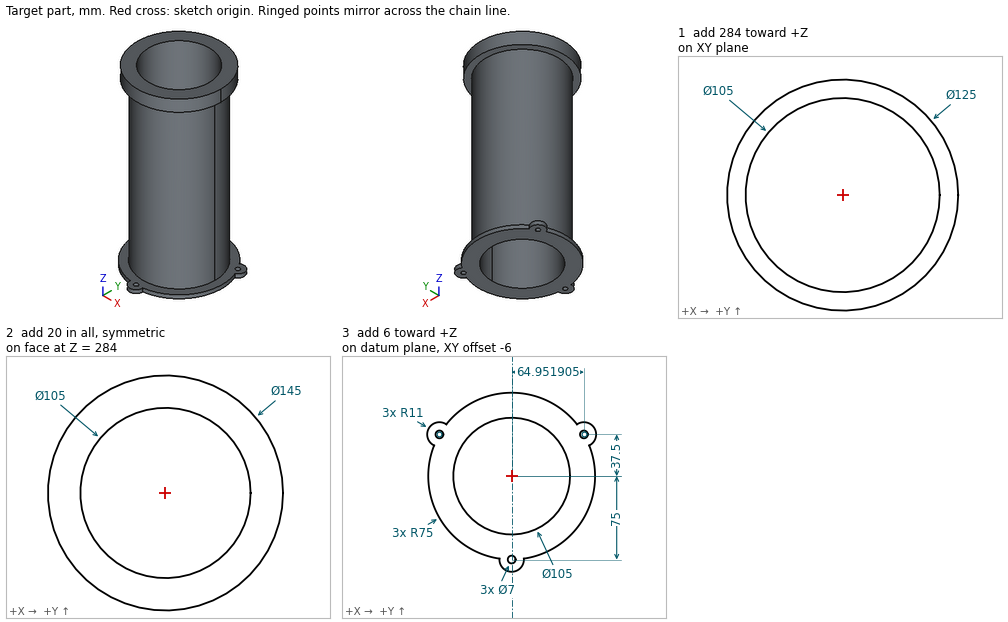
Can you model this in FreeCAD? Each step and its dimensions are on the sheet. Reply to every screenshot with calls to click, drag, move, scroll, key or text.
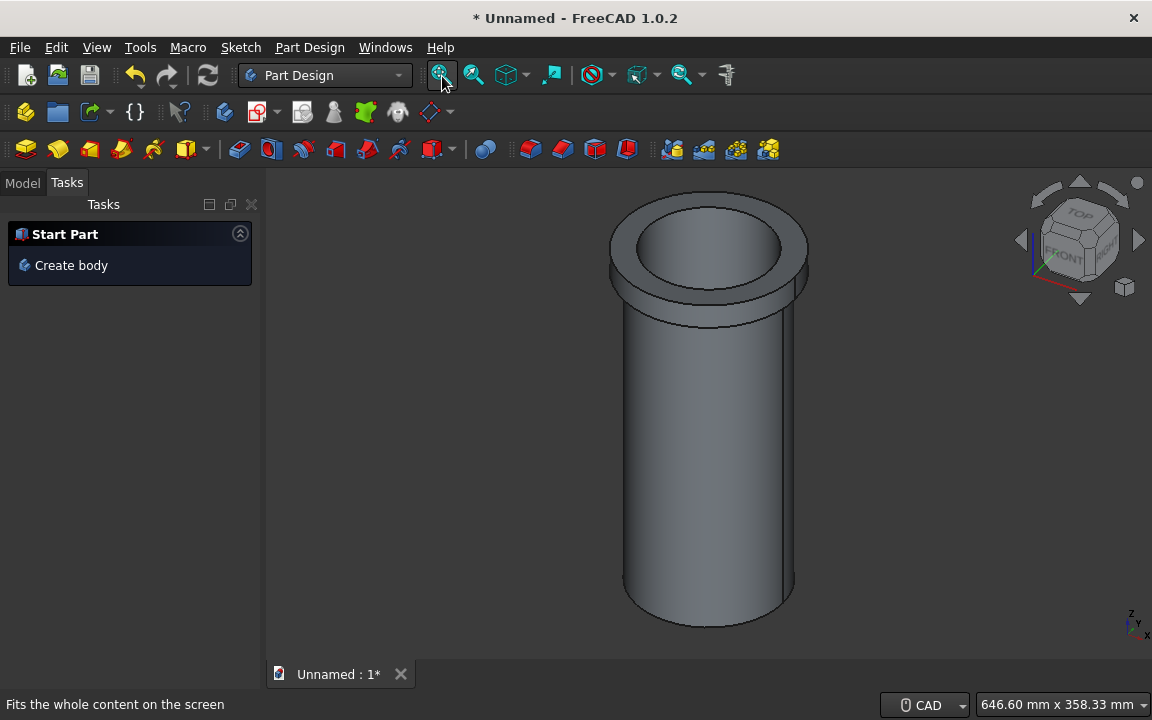
click(23, 182)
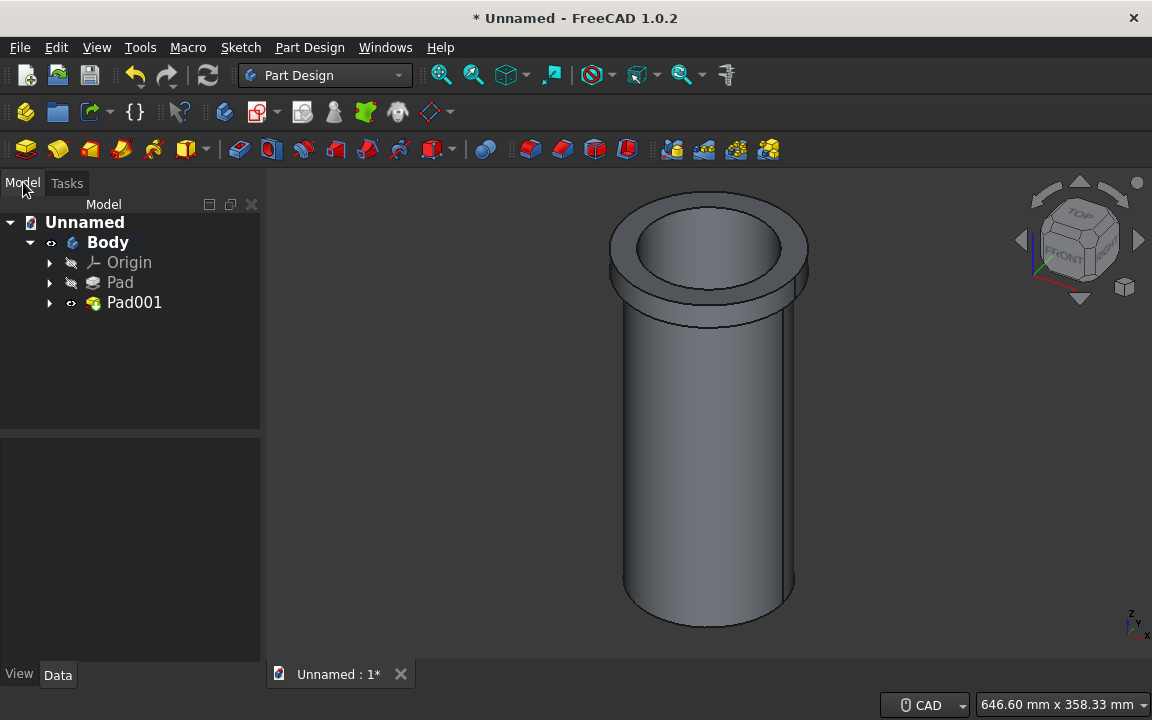
click(50, 263)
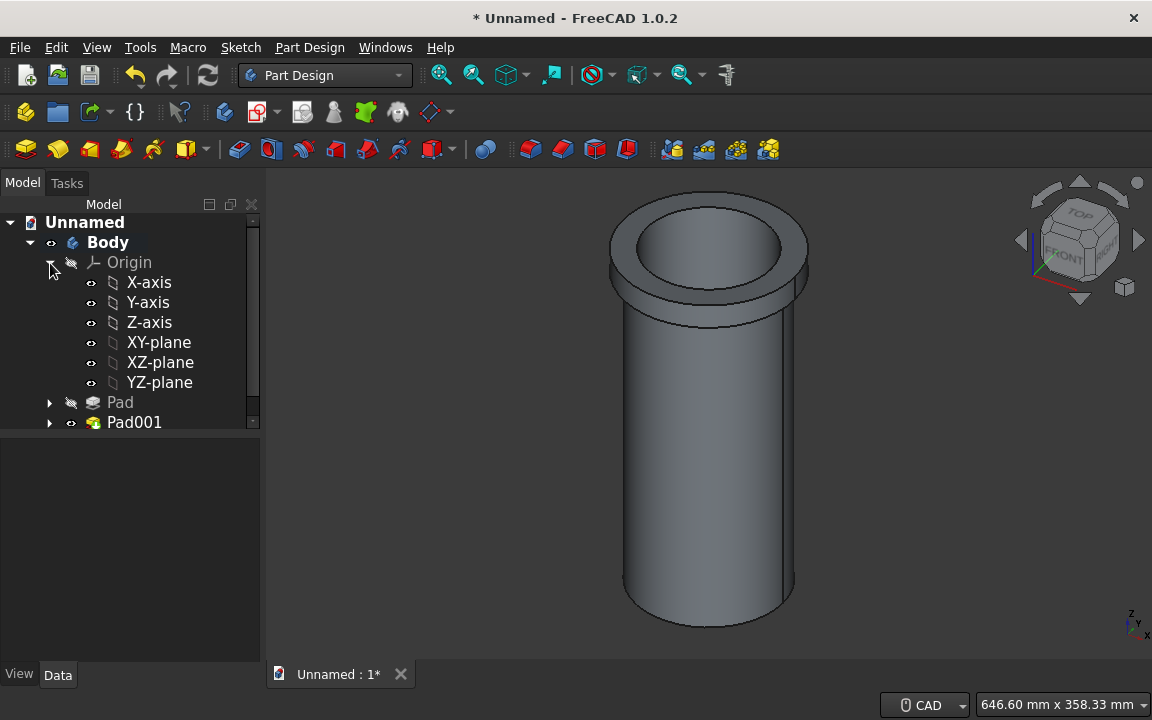
click(136, 343)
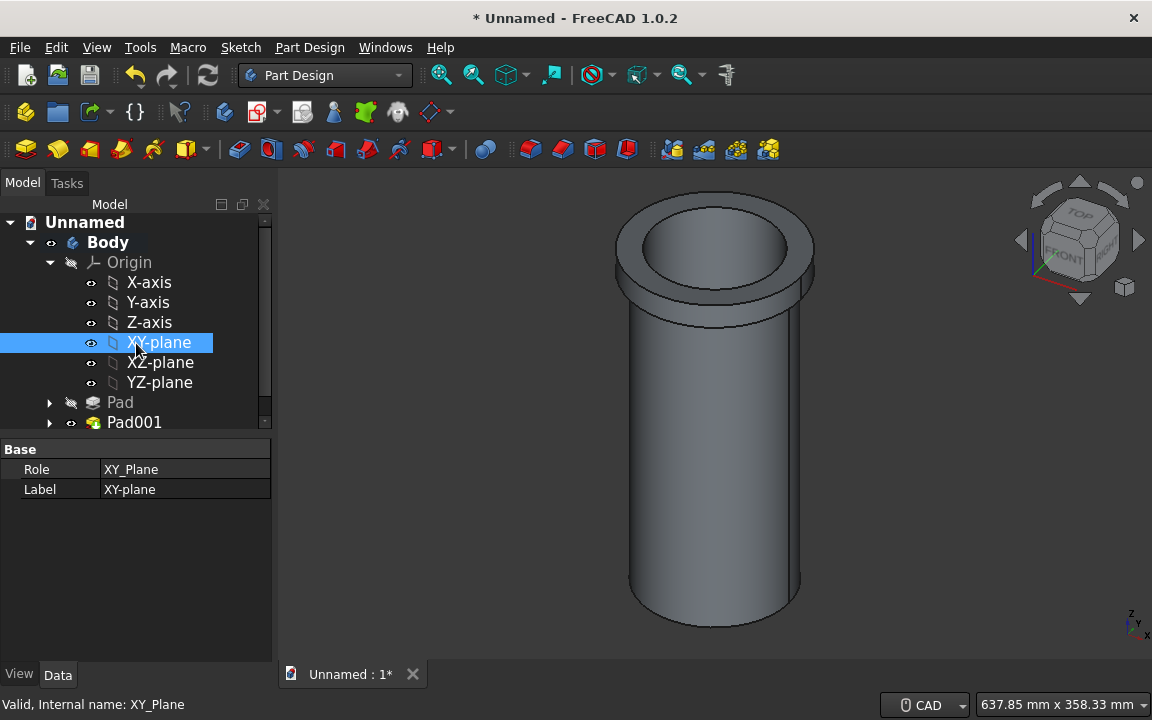
click(430, 112)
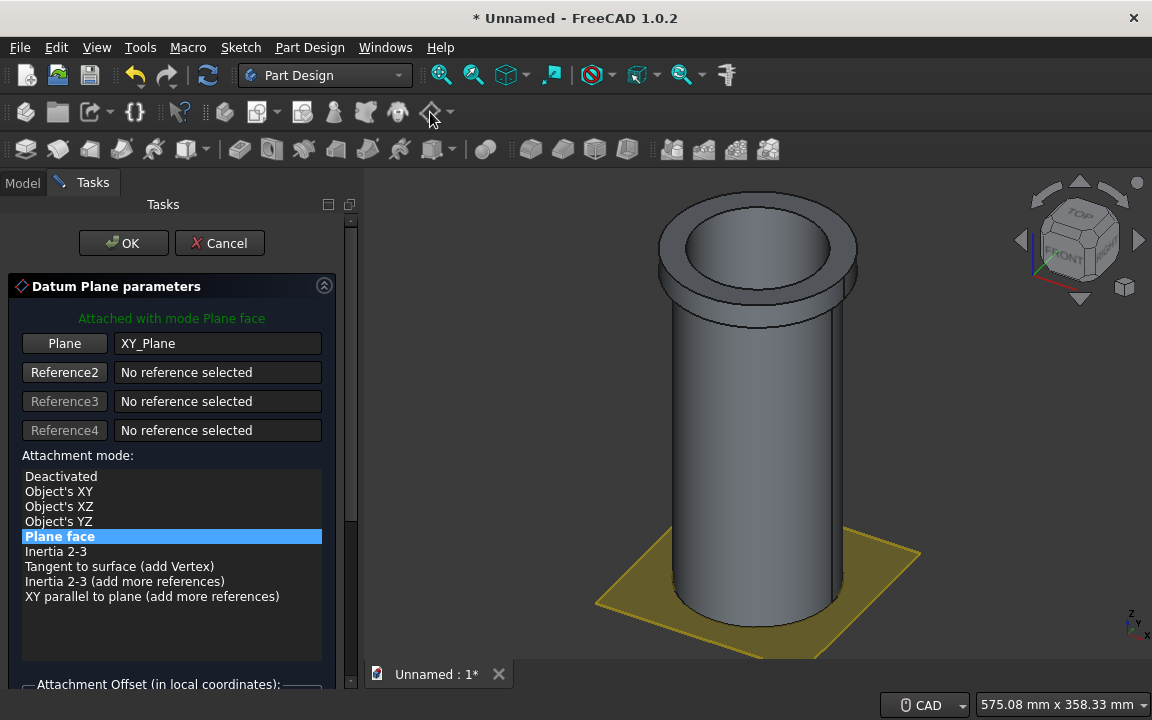
scroll(351, 451, down, 3)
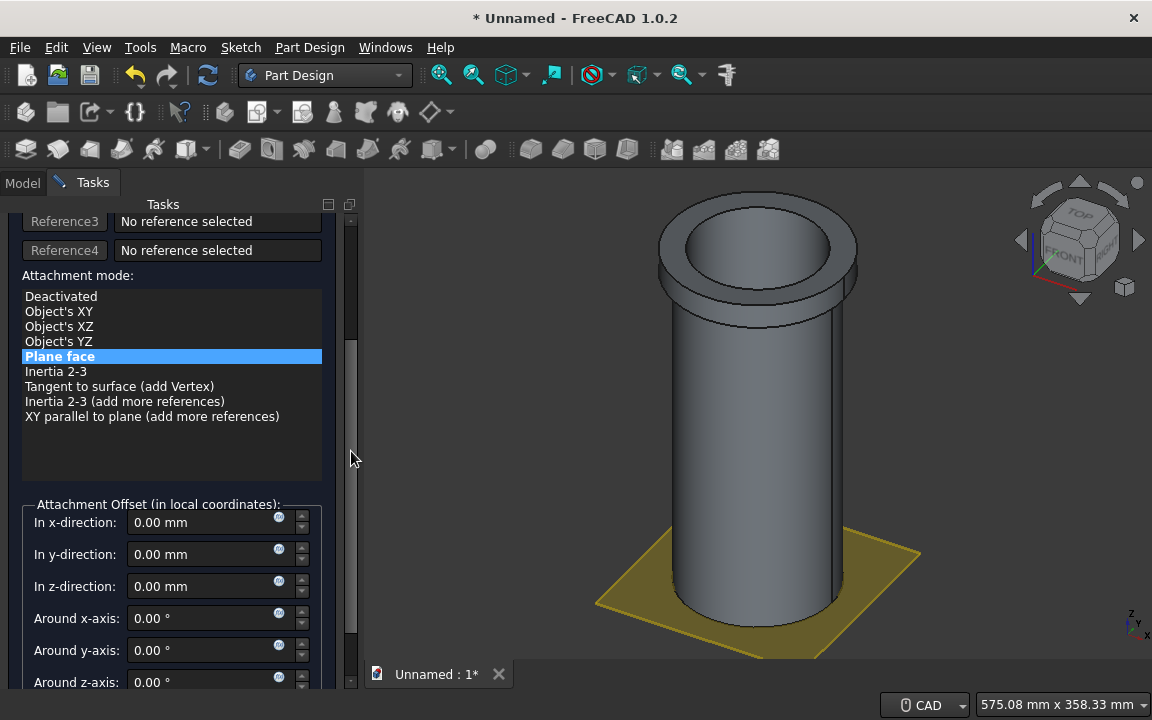
triple_click(210, 586)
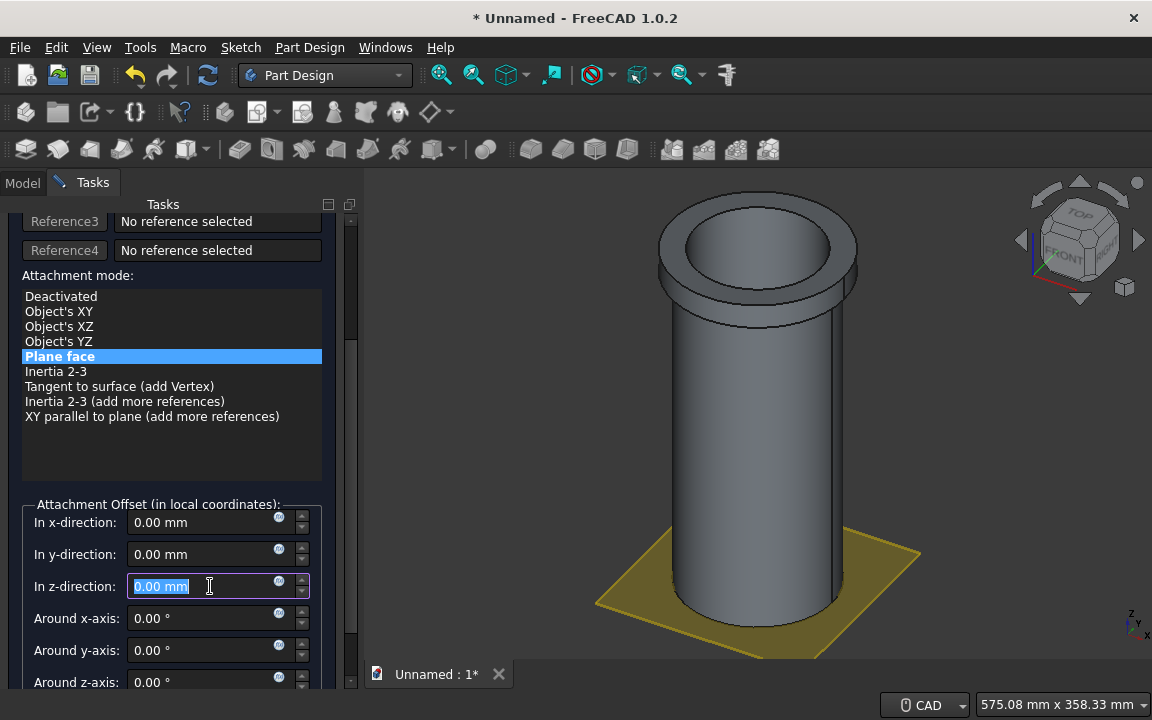
text(-6)
key(Tab)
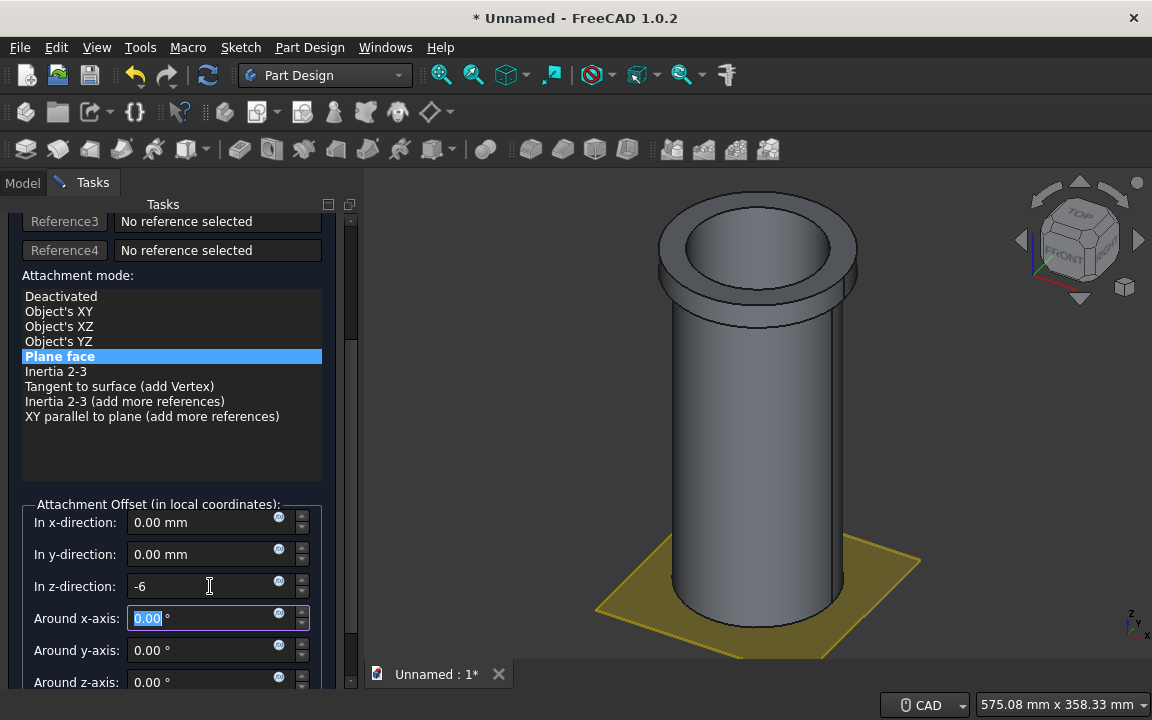
scroll(351, 451, up, 4)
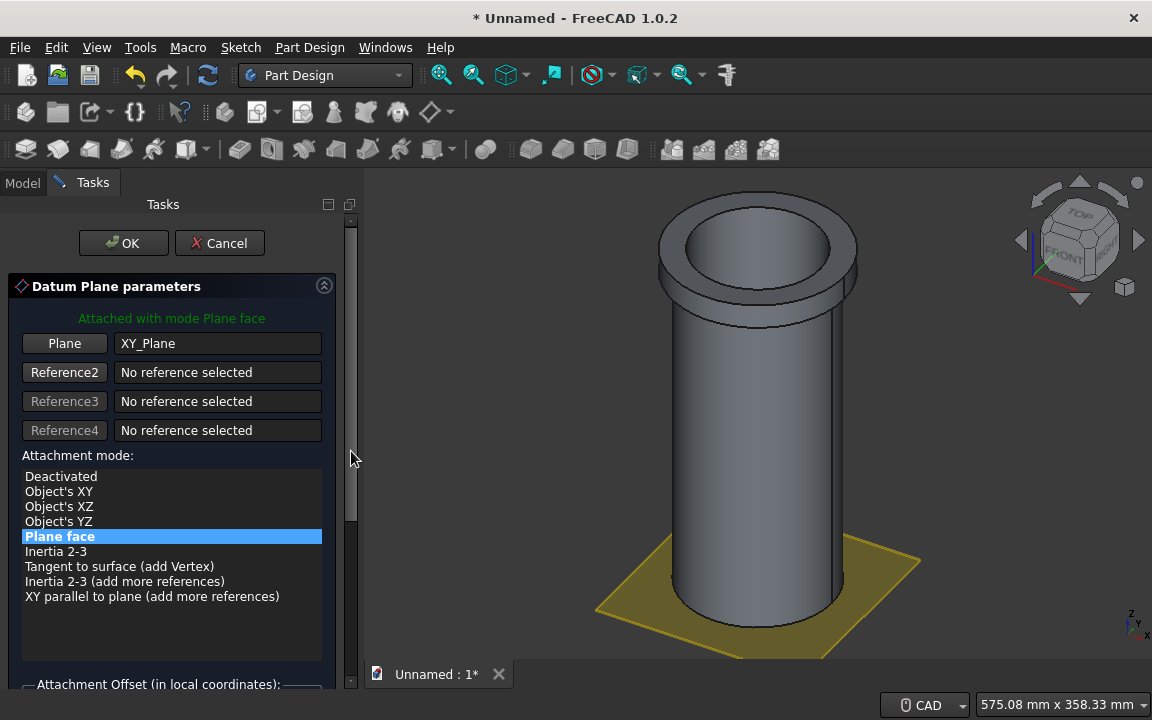
click(124, 243)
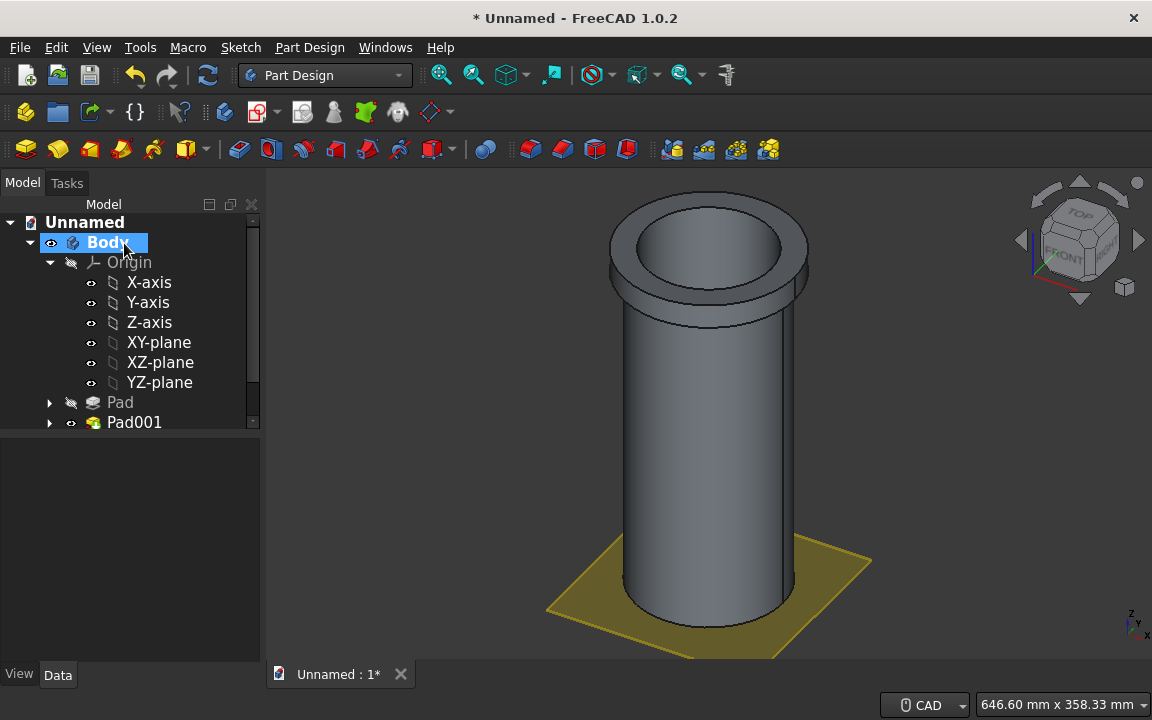
scroll(100, 318, down, 3)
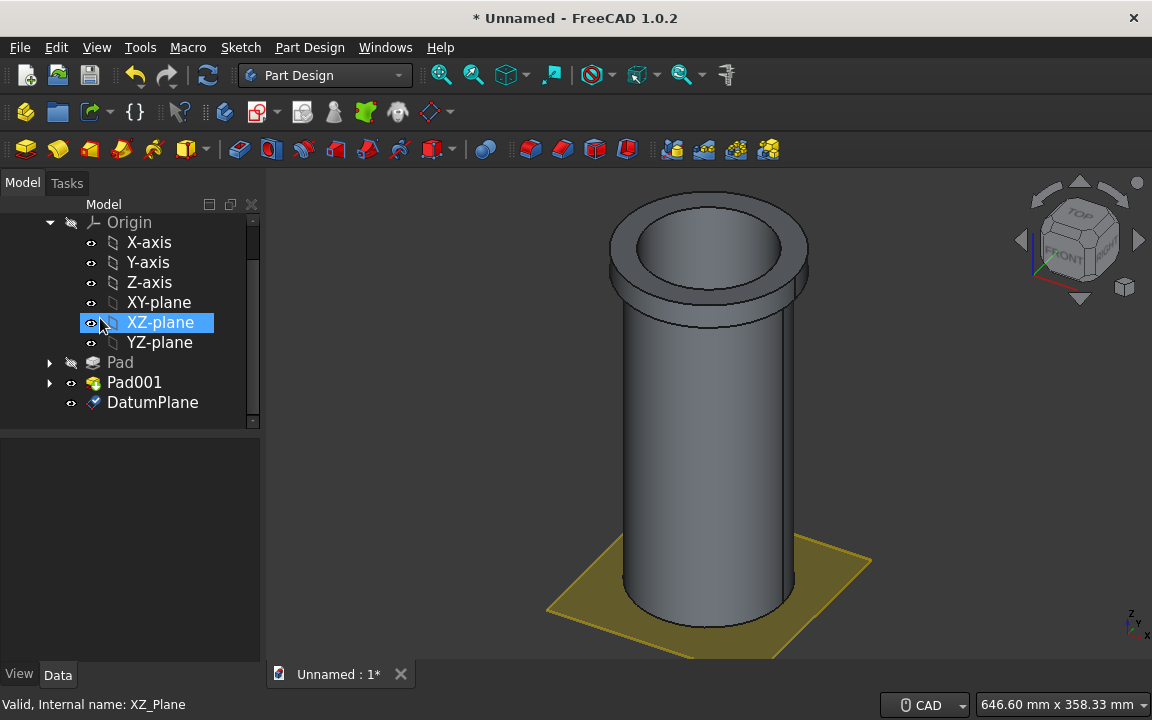
click(116, 403)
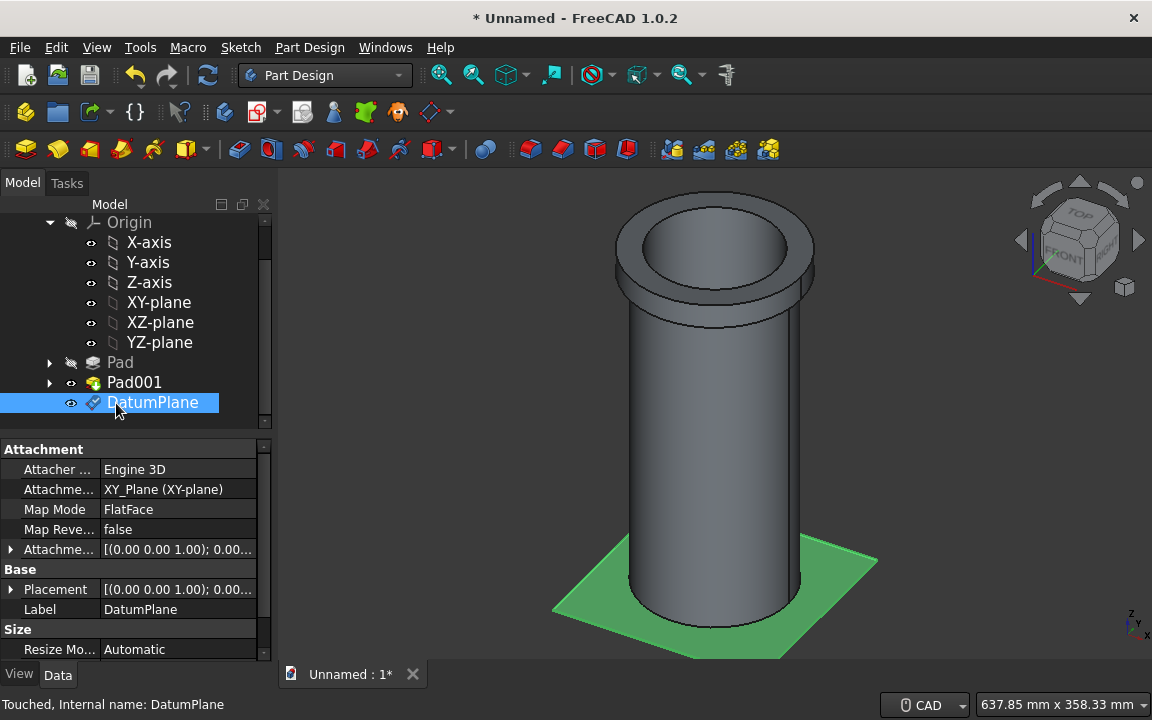
click(258, 112)